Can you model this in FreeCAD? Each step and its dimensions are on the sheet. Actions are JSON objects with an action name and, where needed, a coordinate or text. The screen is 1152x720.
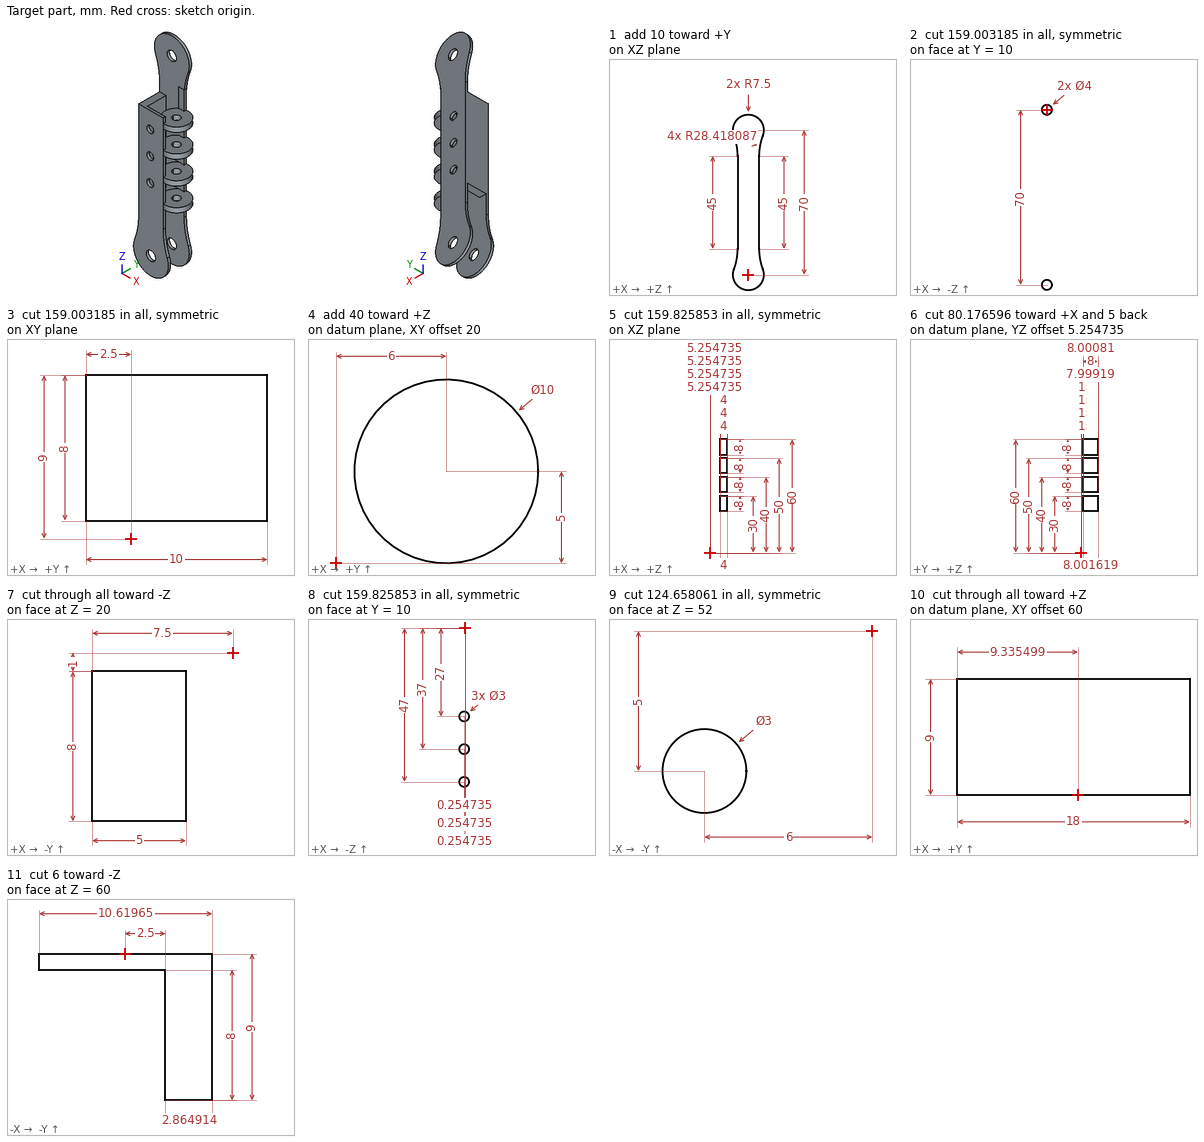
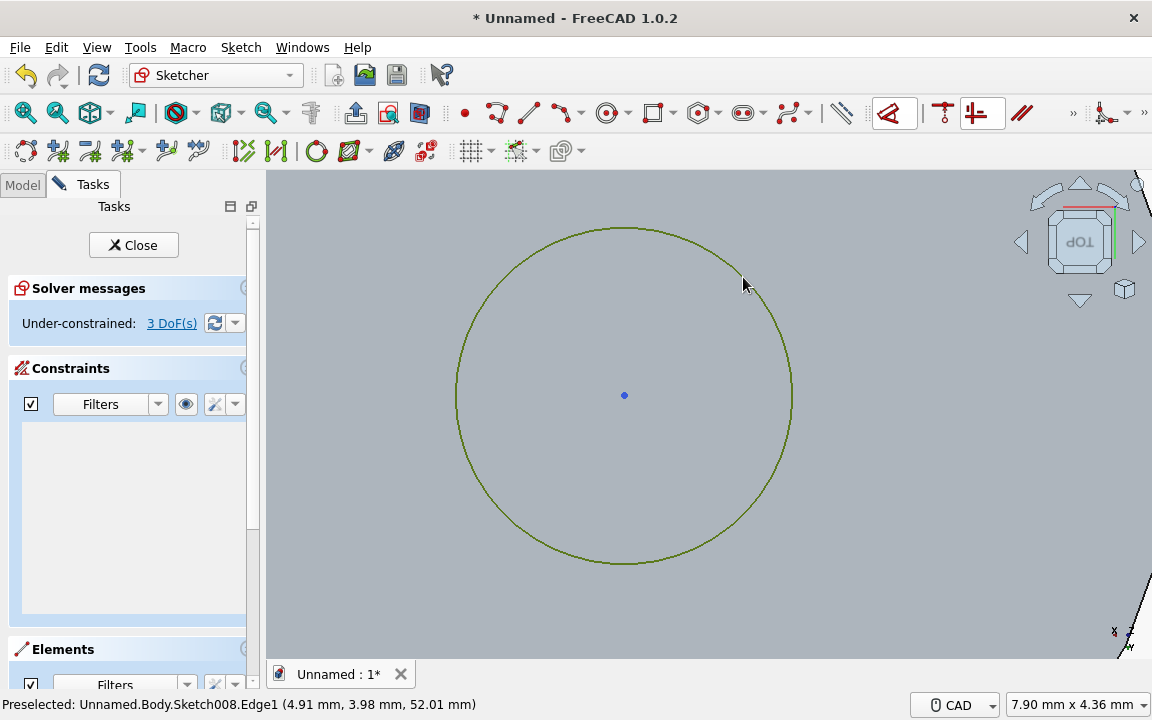
{"action": "key", "text": "k o"}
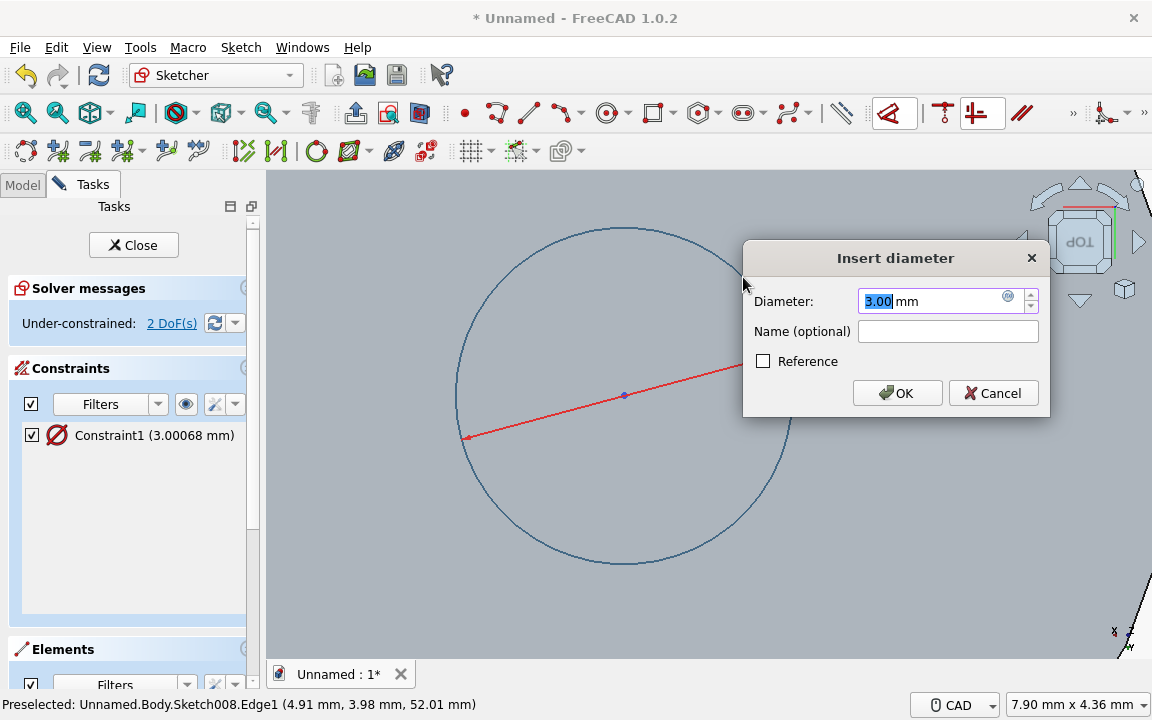
{"action": "type", "text": "3"}
{"action": "key", "text": "Return"}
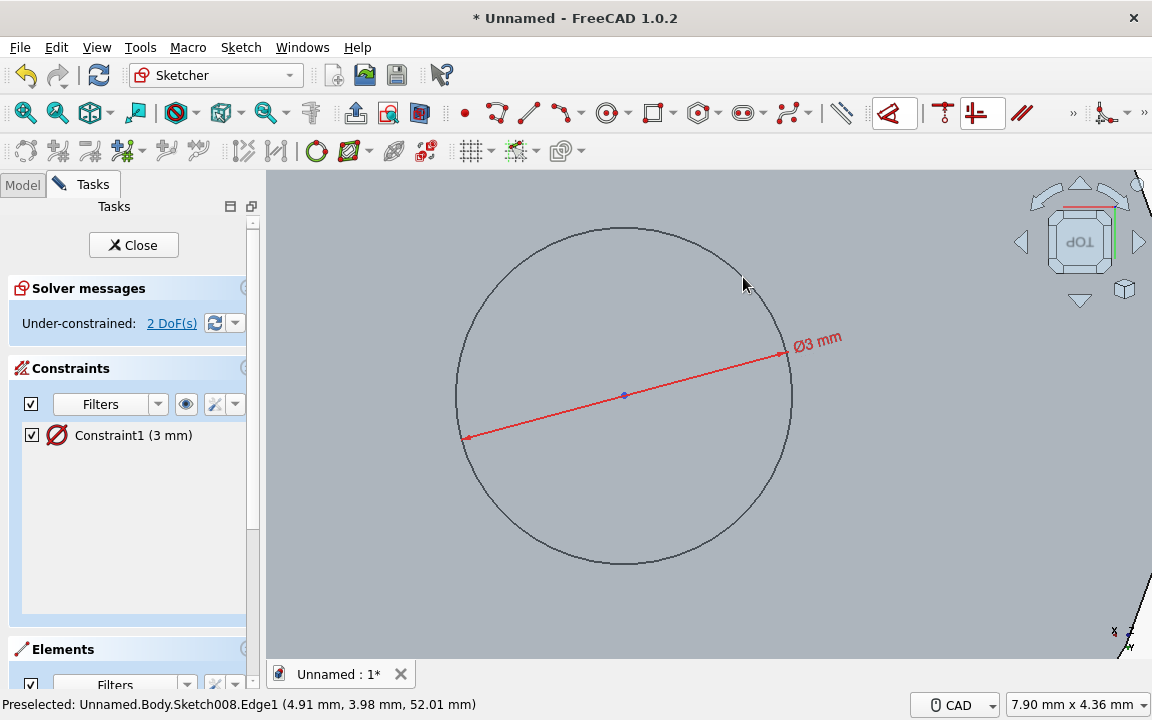
{"action": "left_click", "coordinate": [624, 396]}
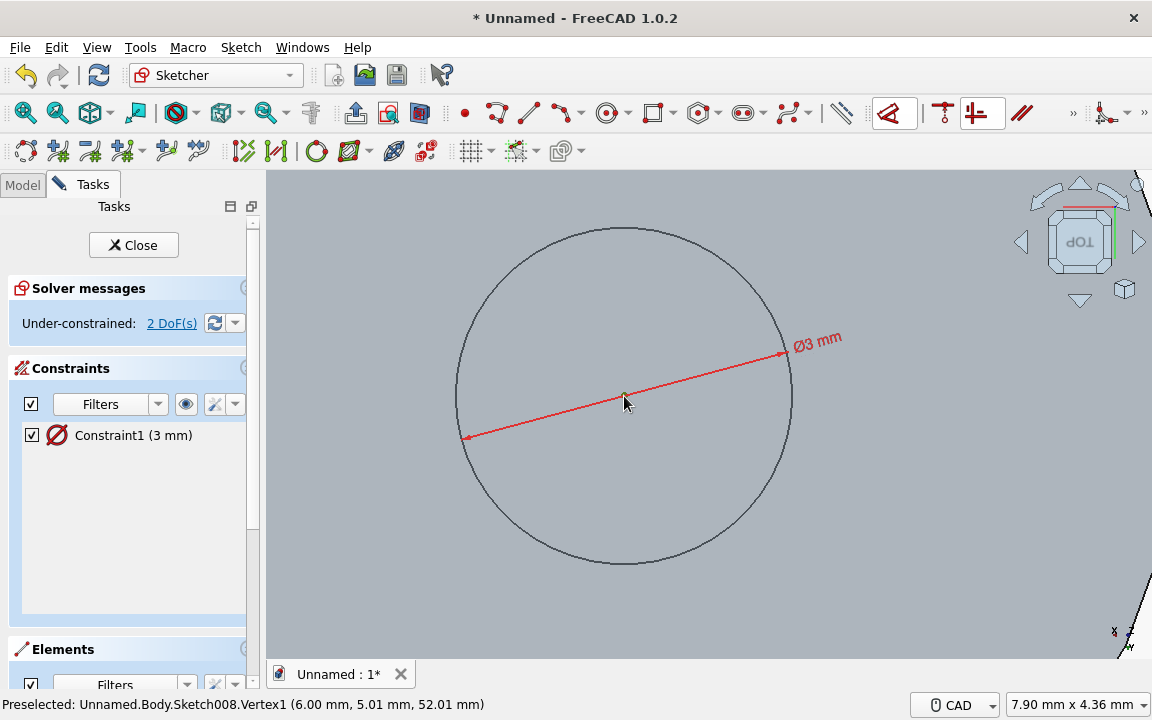
{"action": "key", "text": "l"}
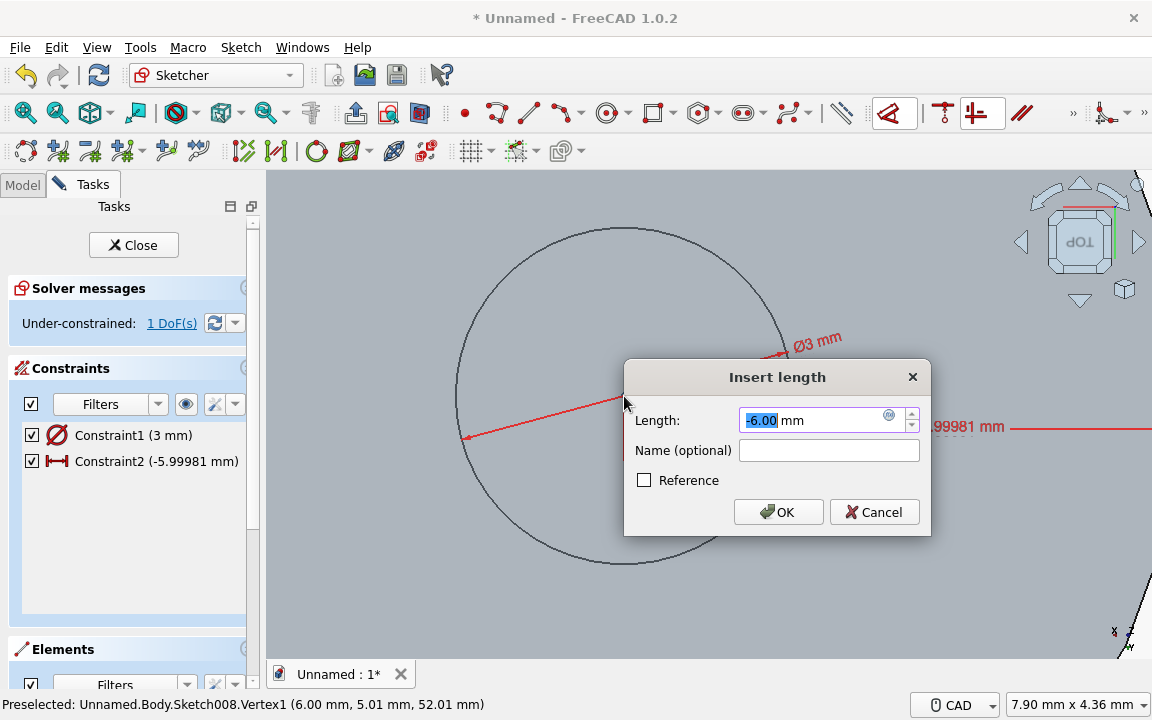
{"action": "type", "text": "-6"}
{"action": "key", "text": "Return"}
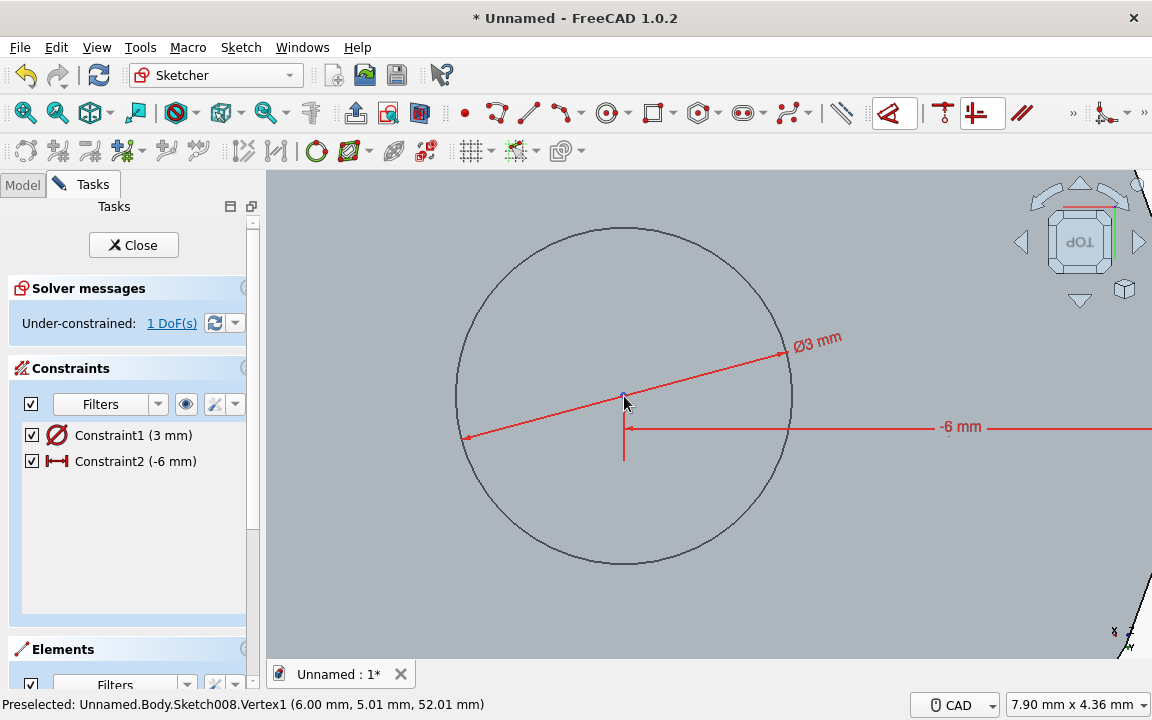
{"action": "left_click", "coordinate": [624, 396]}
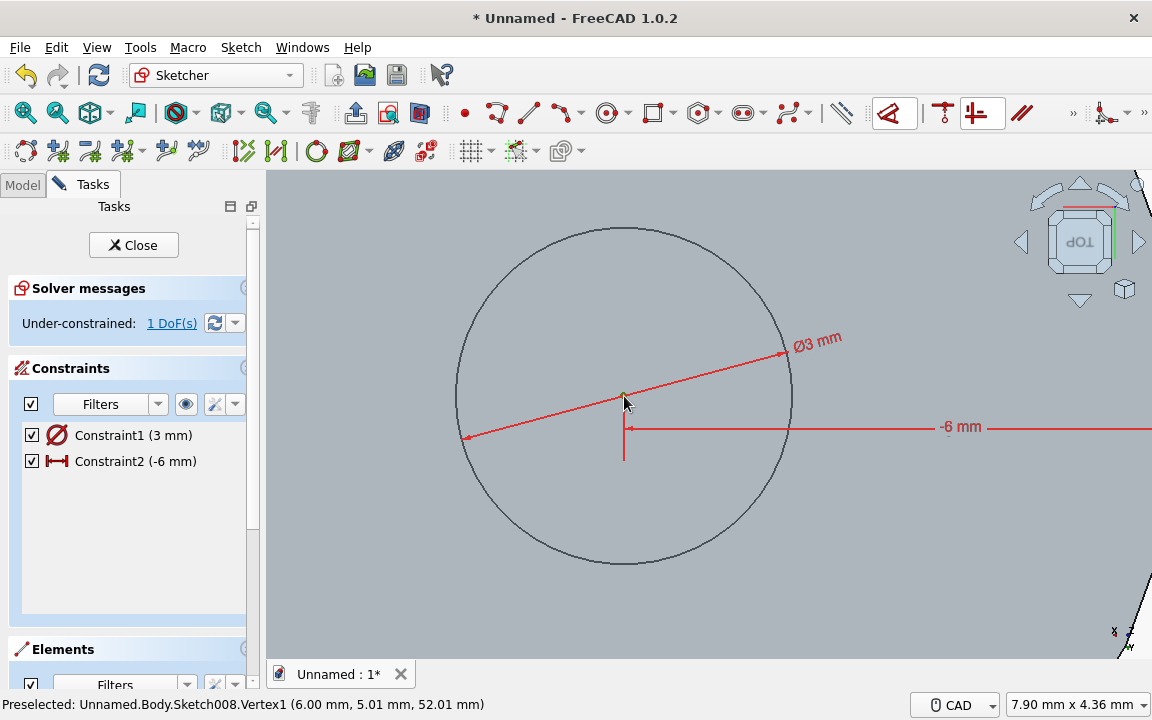
{"action": "key", "text": "i"}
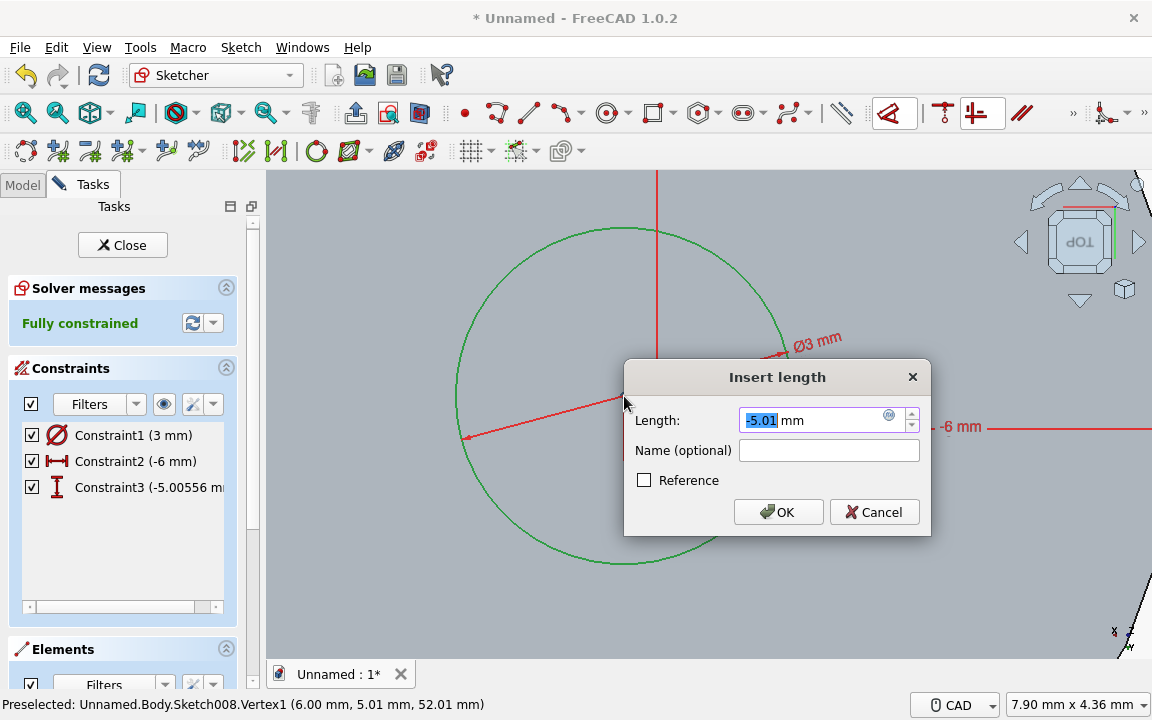
{"action": "type", "text": "-5"}
{"action": "key", "text": "Return"}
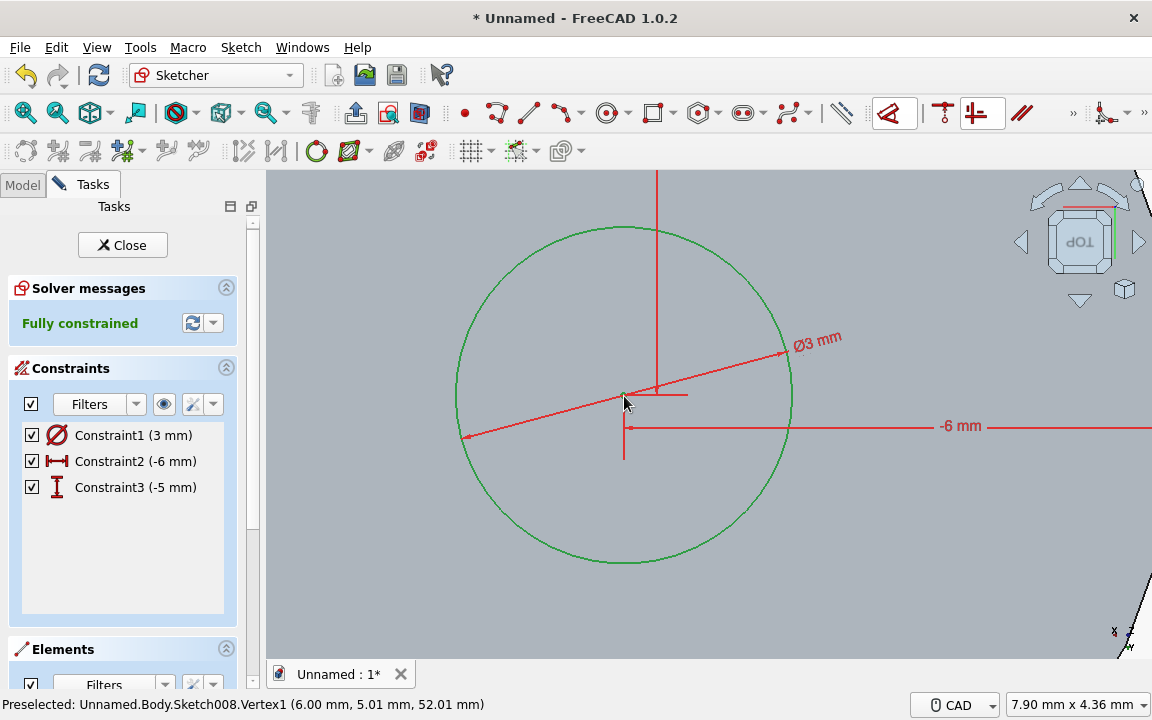
{"action": "left_click", "coordinate": [123, 245]}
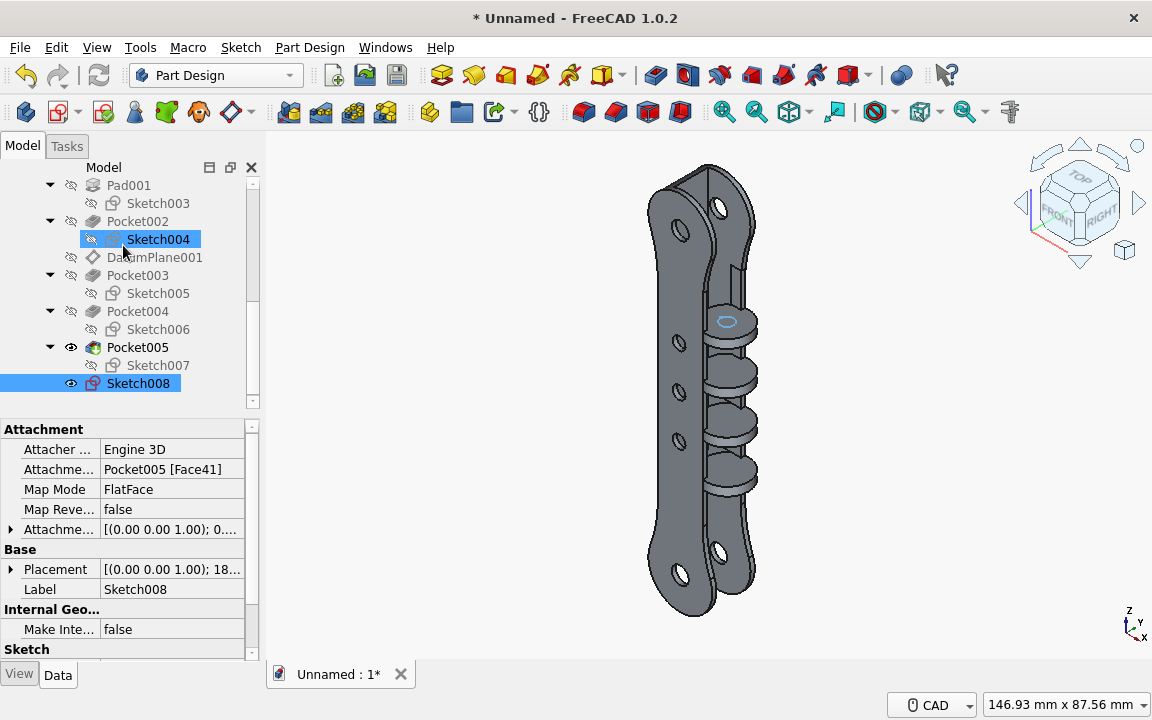
{"action": "left_click", "coordinate": [656, 76]}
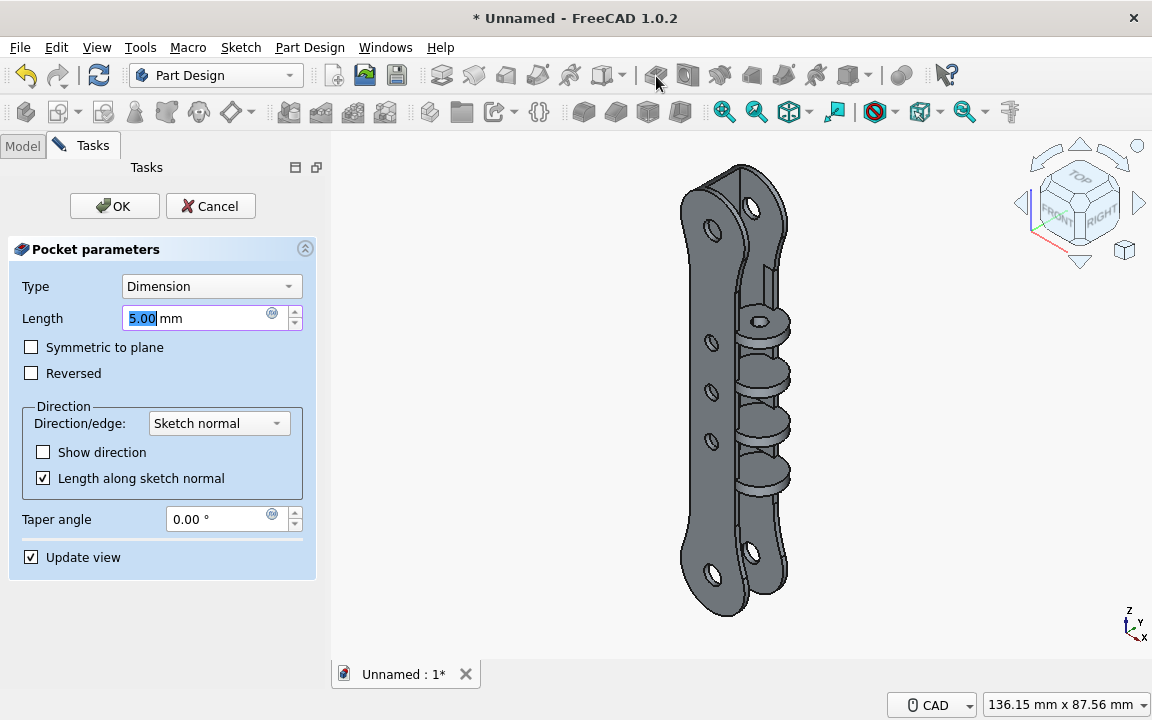
{"action": "type", "text": "124.658061"}
{"action": "key", "text": "Tab"}